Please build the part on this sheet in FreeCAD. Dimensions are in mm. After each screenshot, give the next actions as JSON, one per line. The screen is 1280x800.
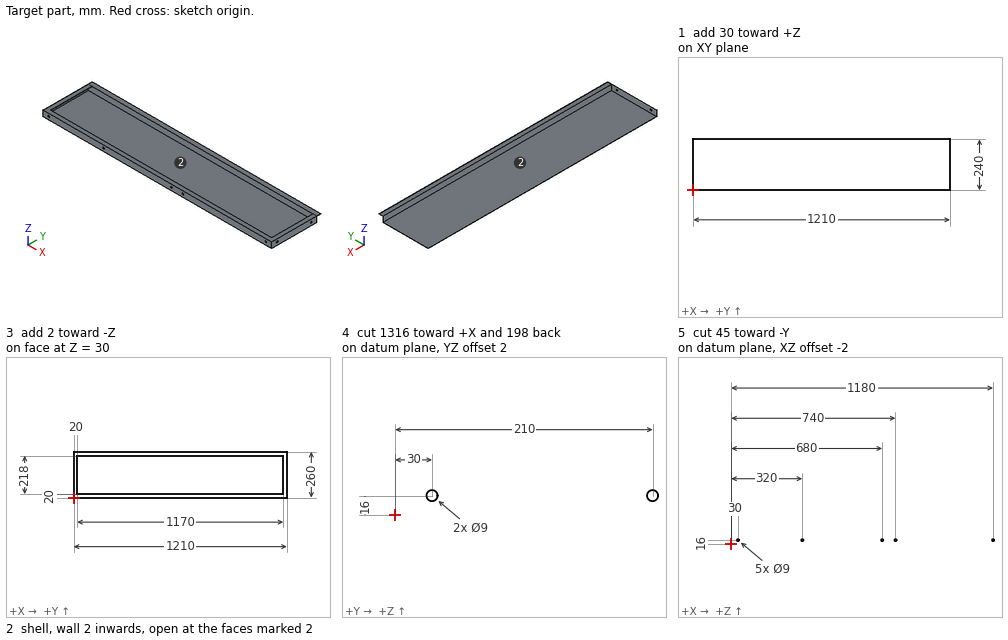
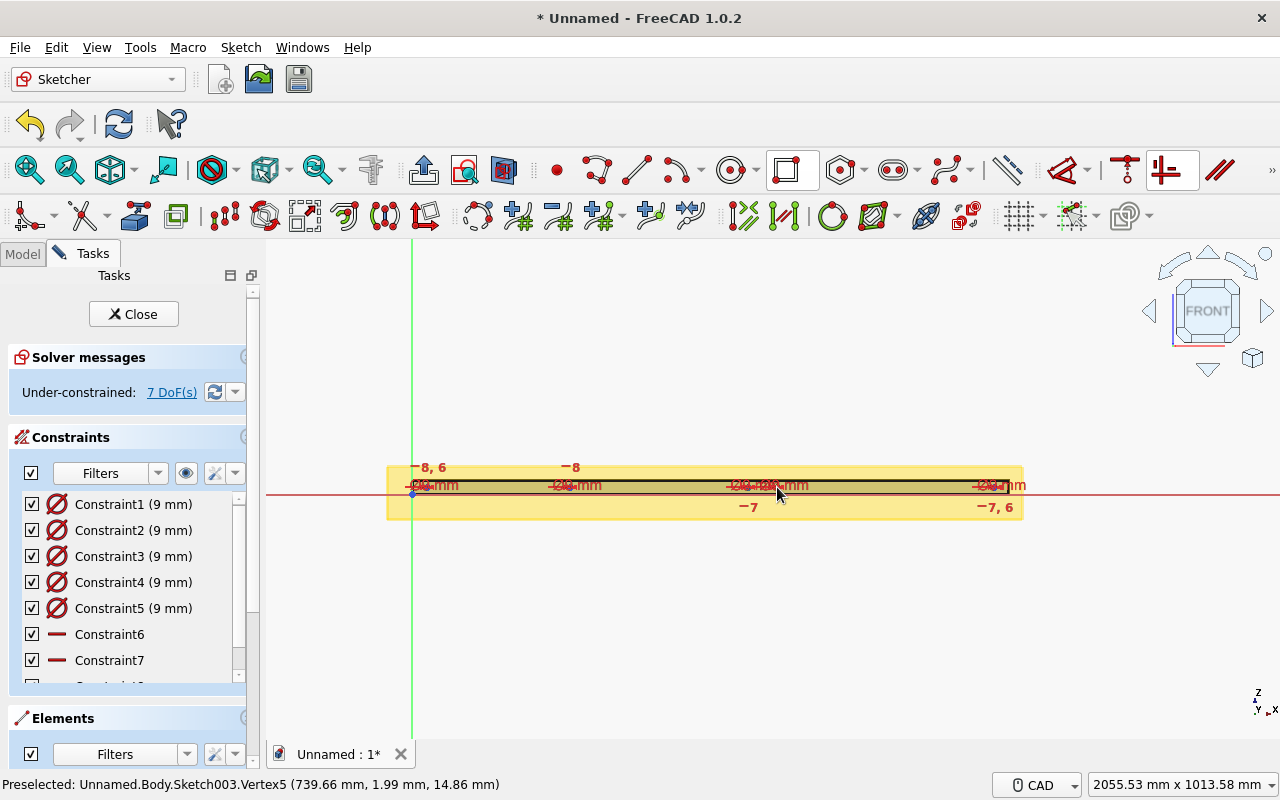
{"action": "left_click", "coordinate": [1194, 170]}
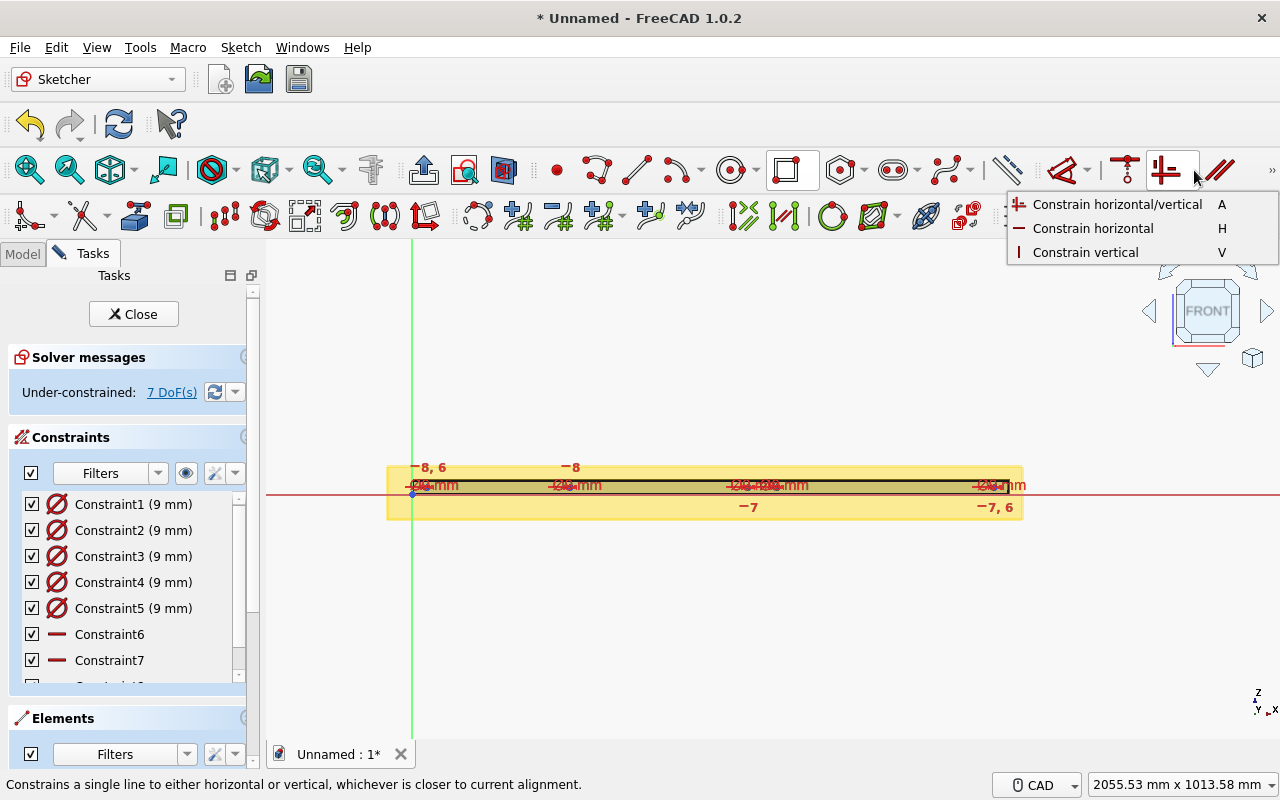
{"action": "left_click", "coordinate": [1143, 228]}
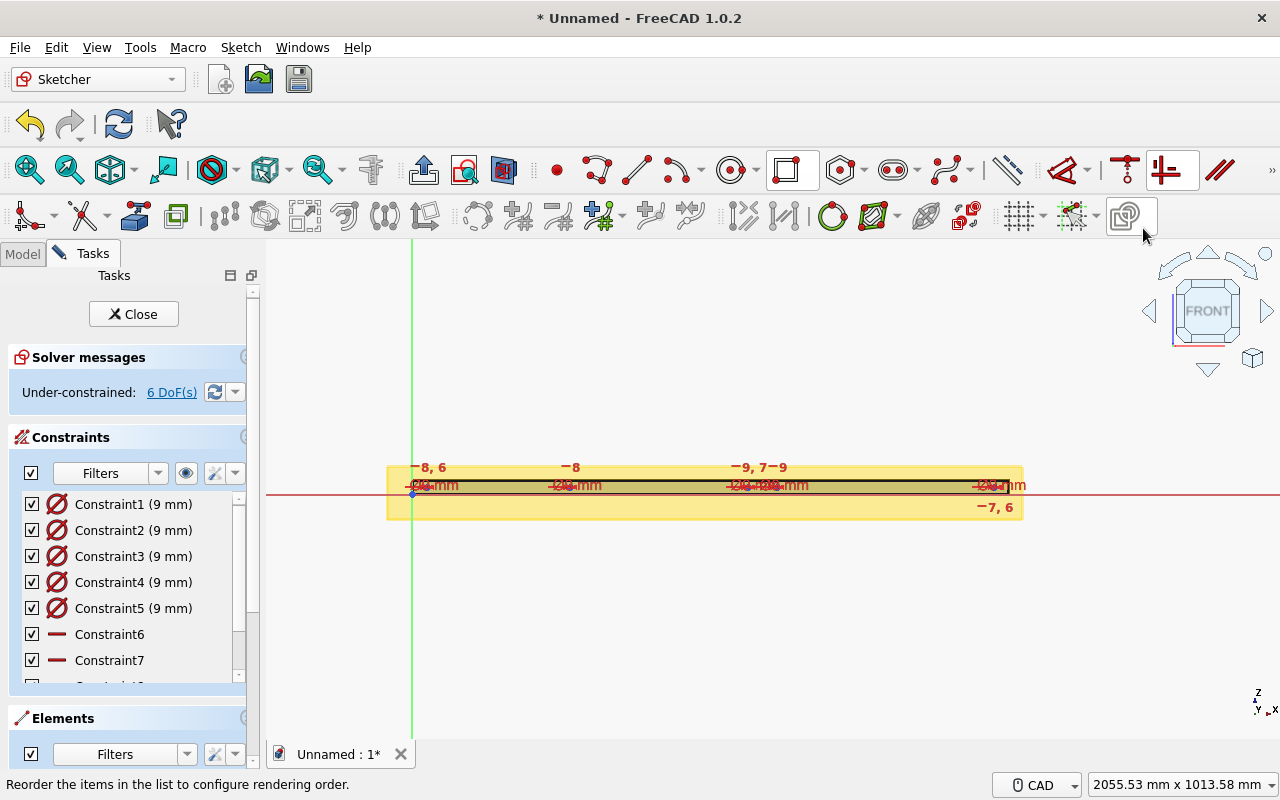
{"action": "left_click", "coordinate": [1062, 170]}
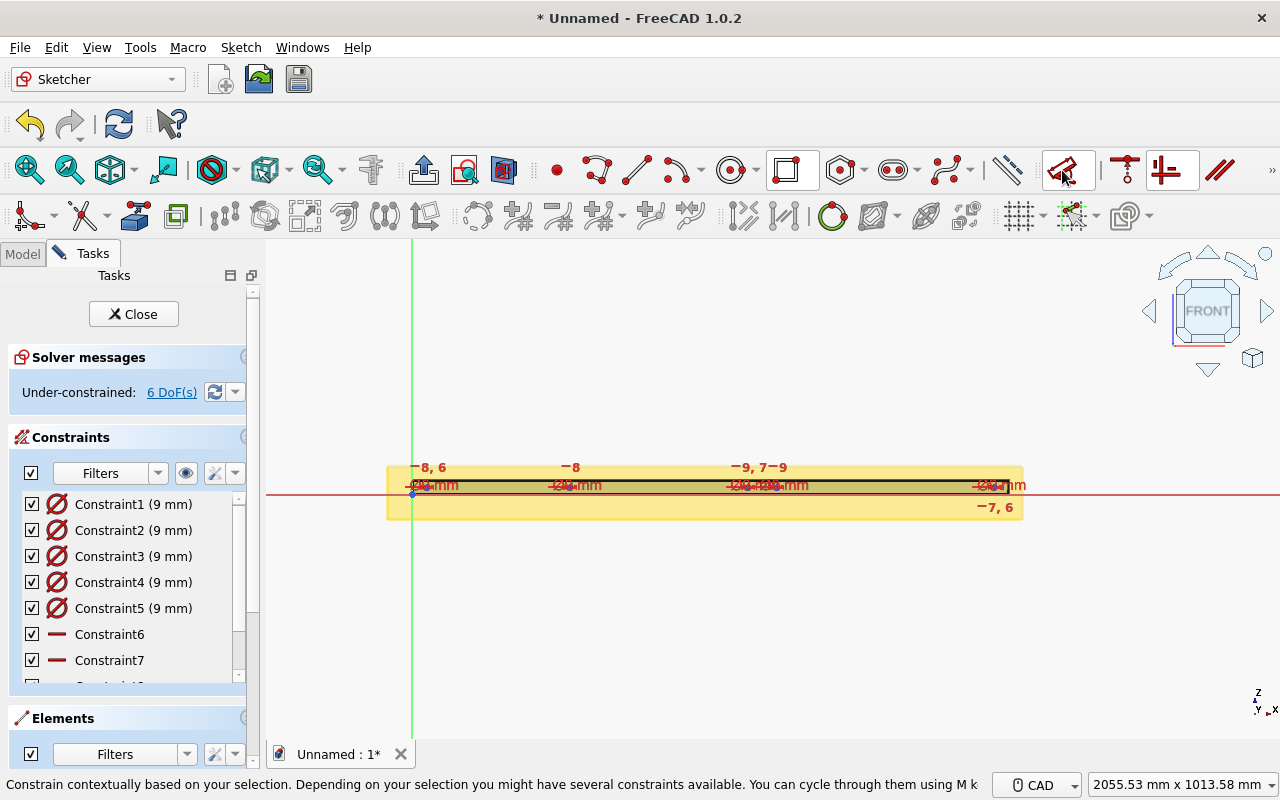
{"action": "scroll", "coordinate": [427, 487], "scroll_direction": "up", "scroll_amount": 5}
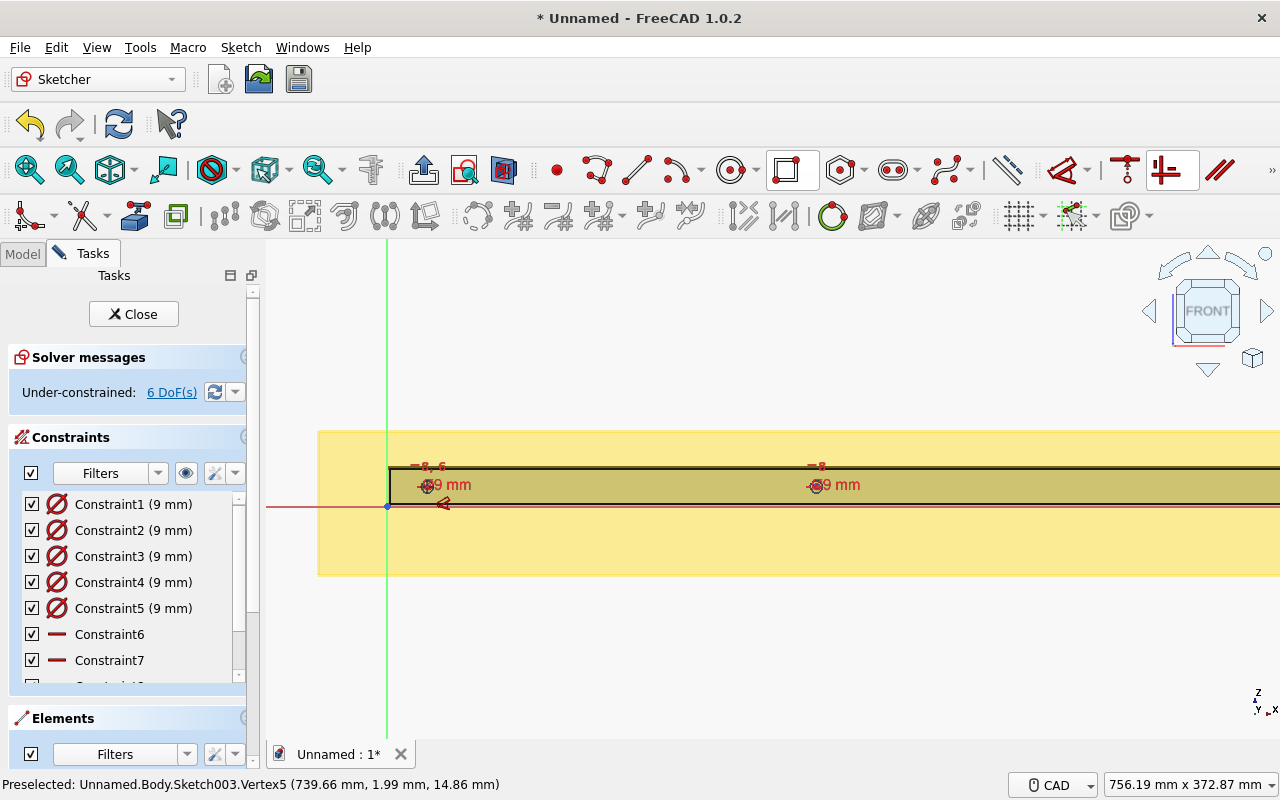
{"action": "left_click", "coordinate": [427, 487]}
{"action": "left_click", "coordinate": [407, 541]}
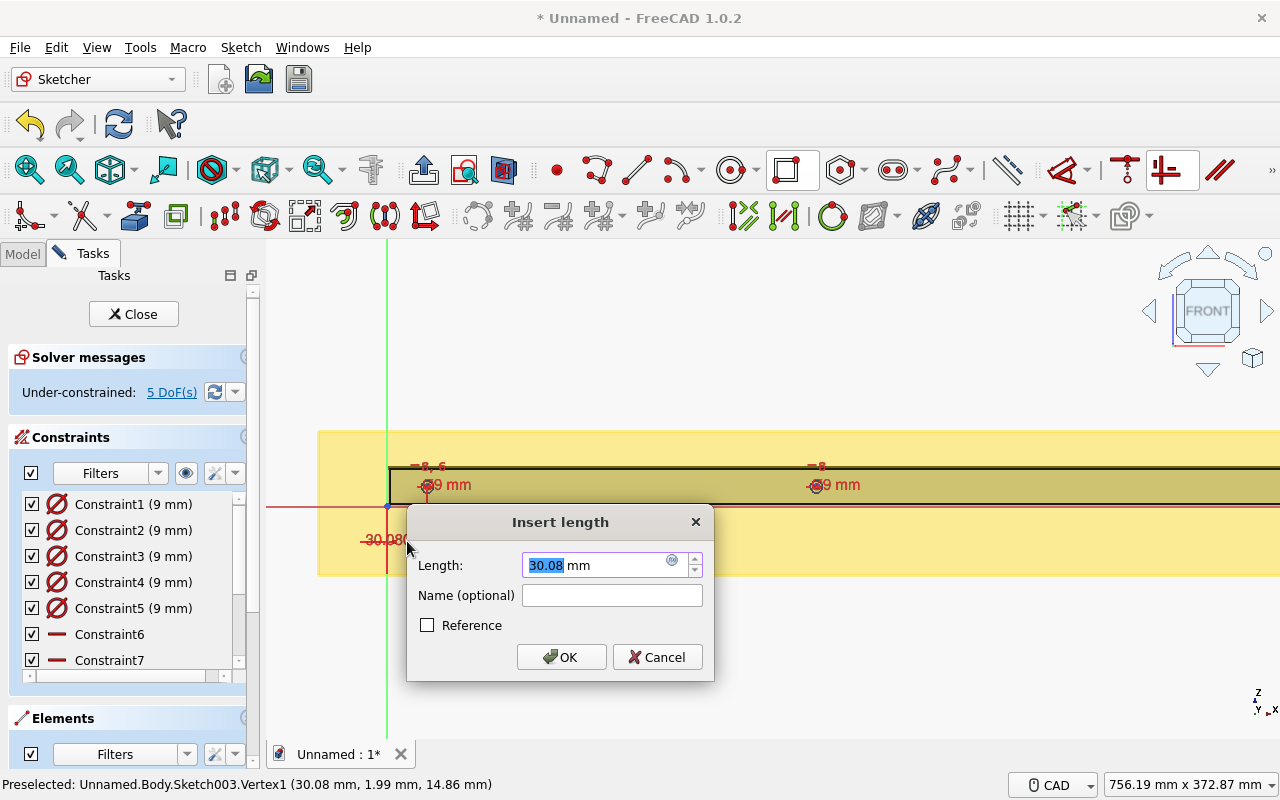
{"action": "type", "text": "30"}
{"action": "key", "text": "Return"}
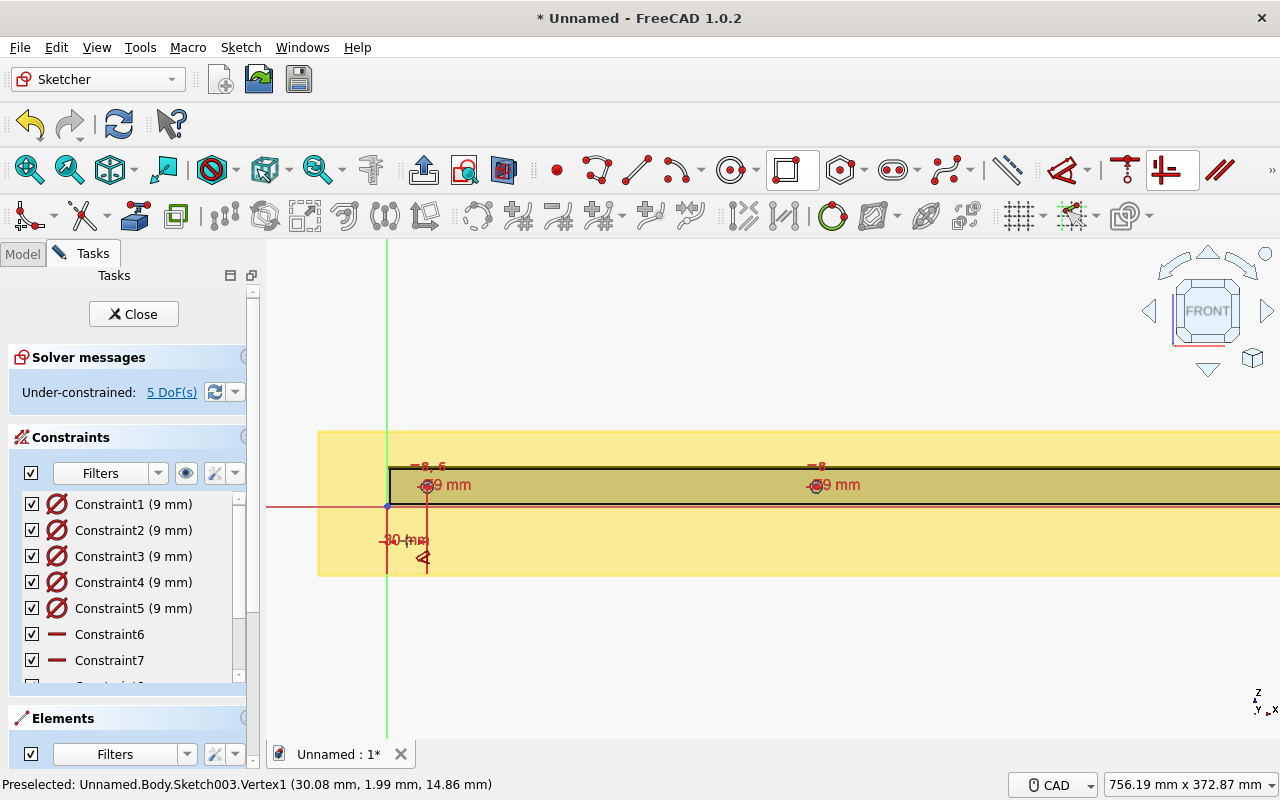
{"action": "scroll", "coordinate": [427, 487], "scroll_direction": "up", "scroll_amount": 4}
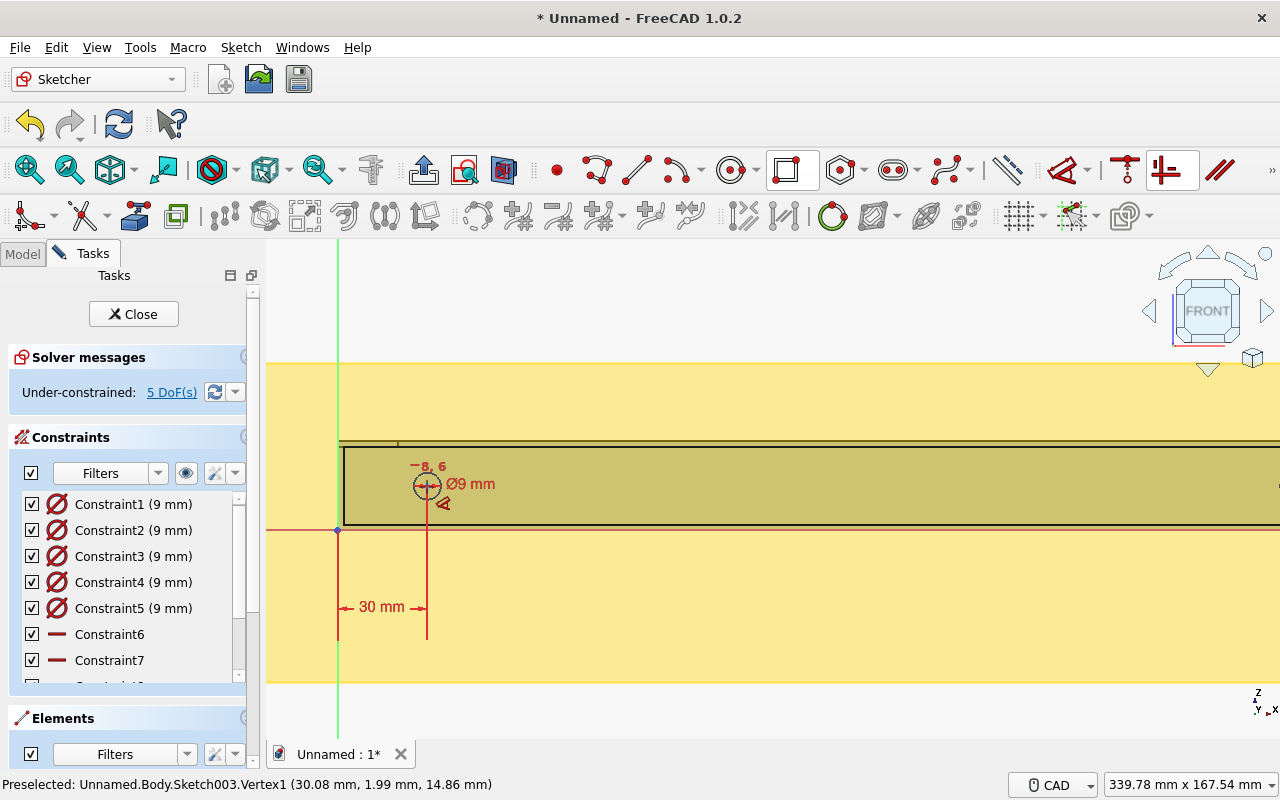
{"action": "left_click", "coordinate": [427, 486]}
{"action": "left_click", "coordinate": [304, 508]}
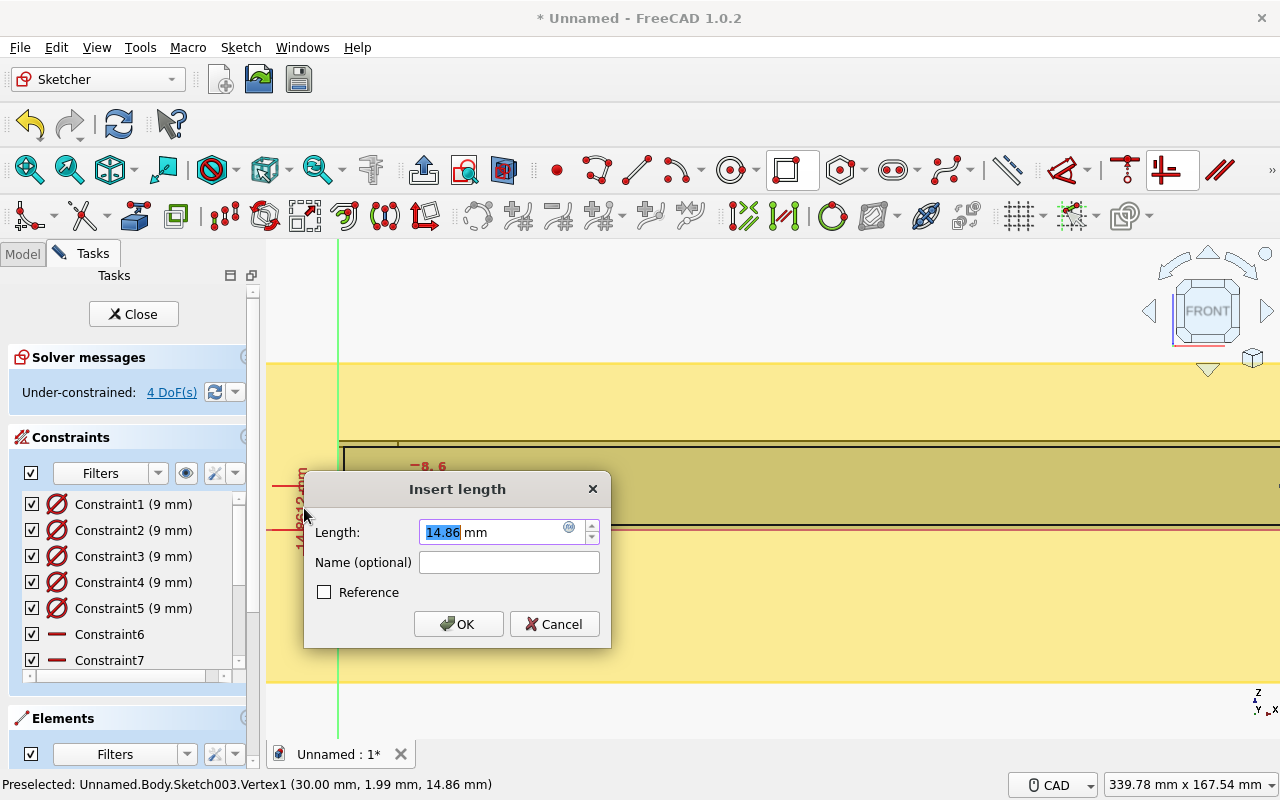
{"action": "type", "text": "16"}
{"action": "key", "text": "Return"}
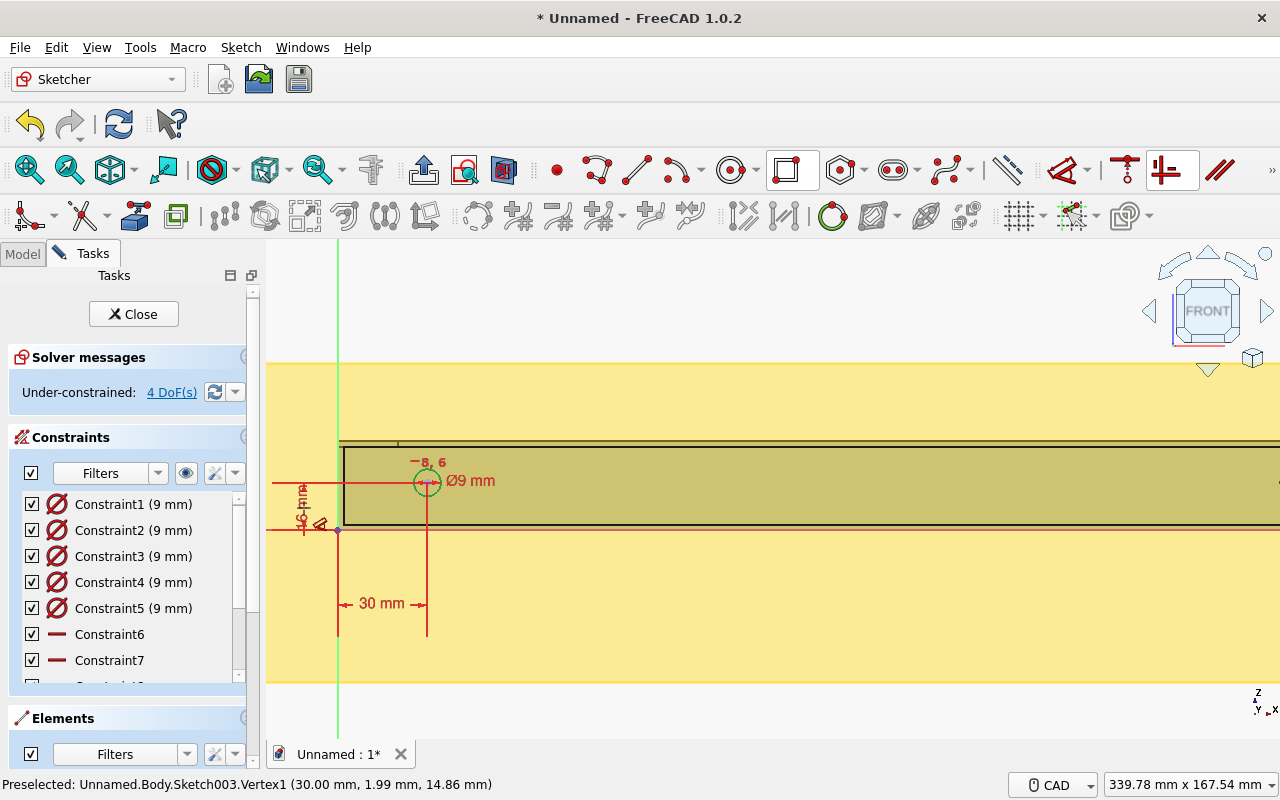
{"action": "scroll", "coordinate": [427, 487], "scroll_direction": "down", "scroll_amount": 9}